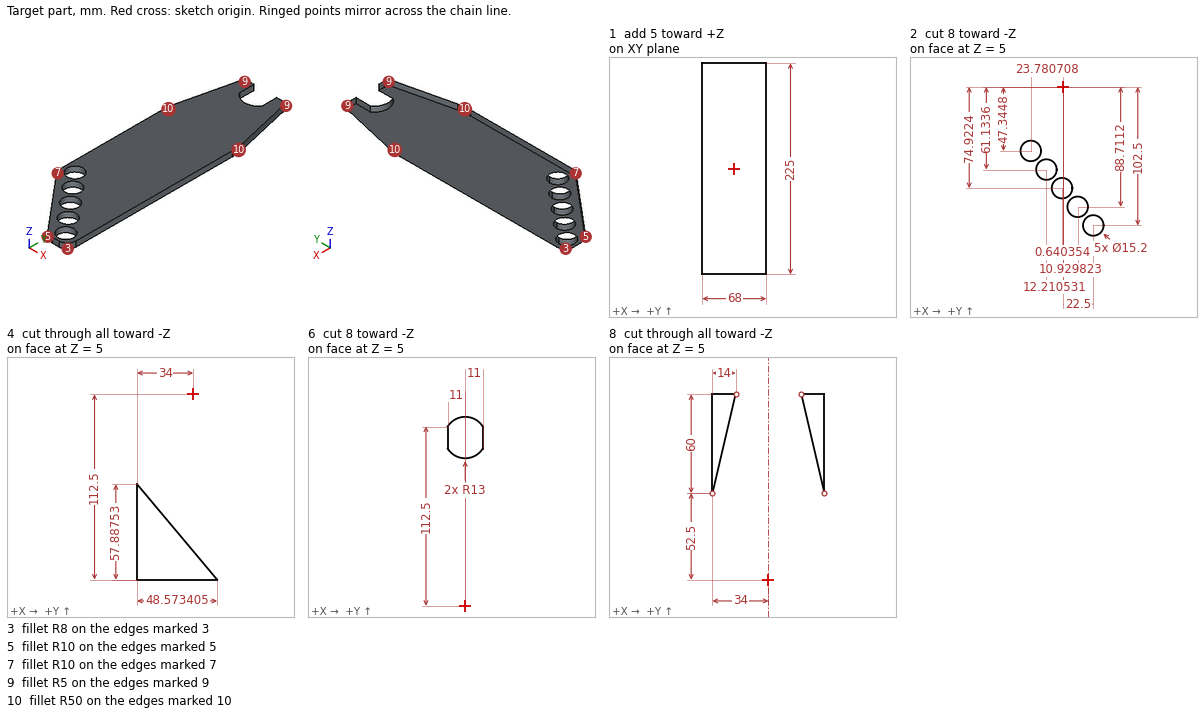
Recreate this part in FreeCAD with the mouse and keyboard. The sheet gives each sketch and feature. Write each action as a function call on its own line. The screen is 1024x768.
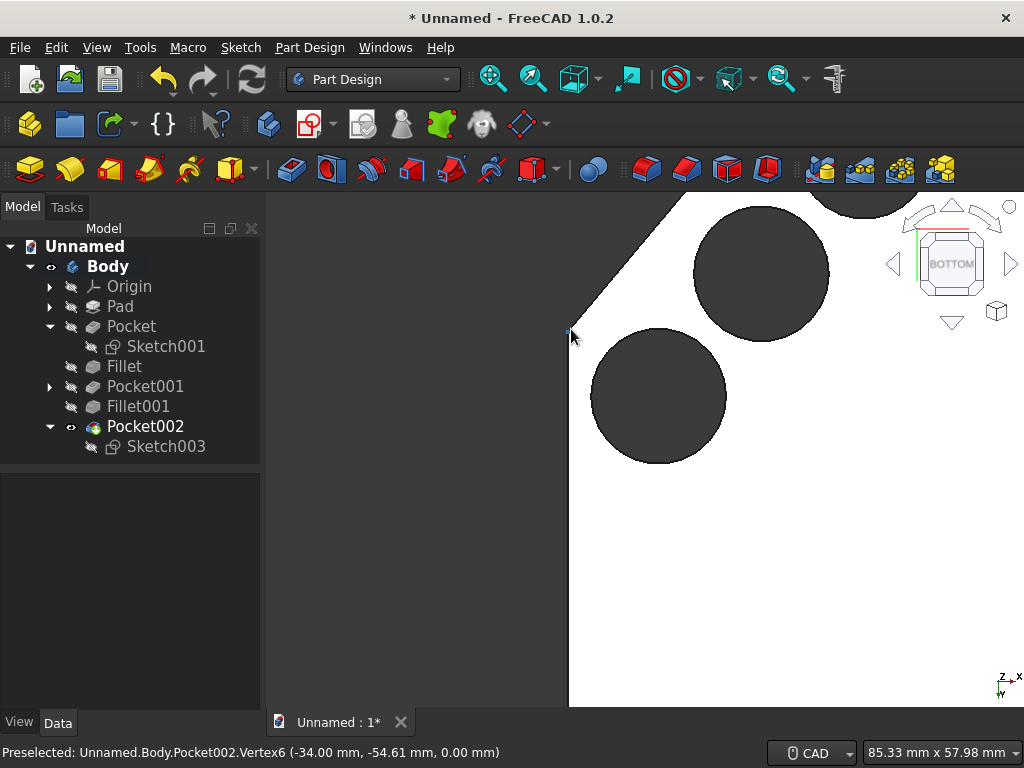
key(v)
key(f)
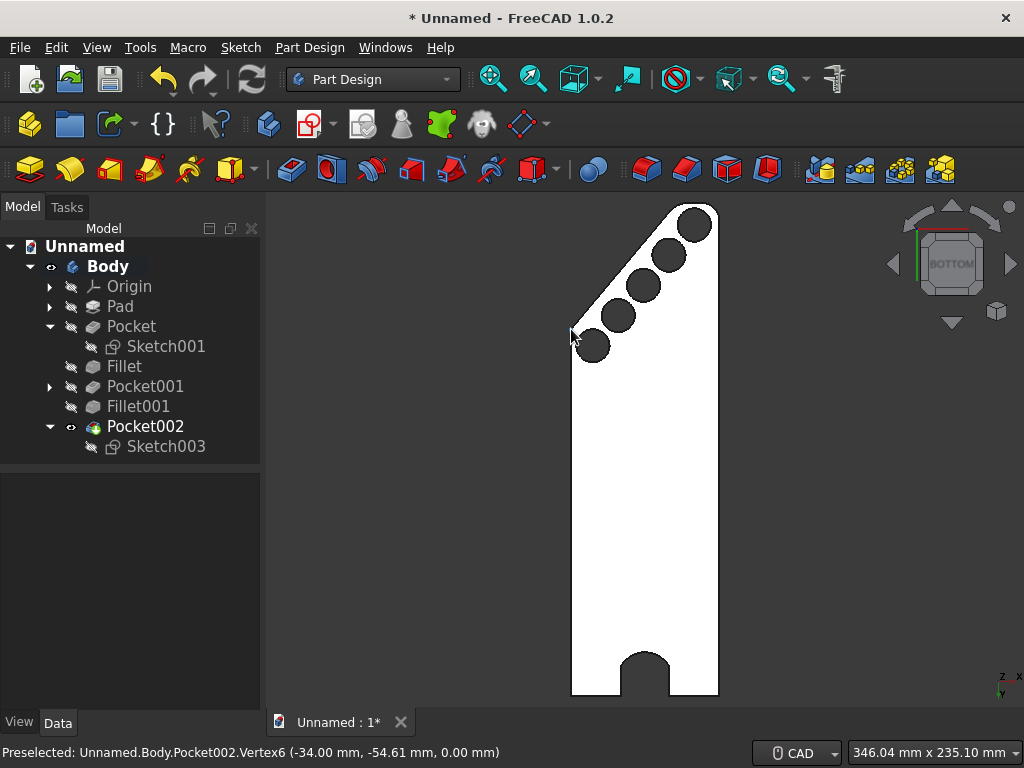
key(4)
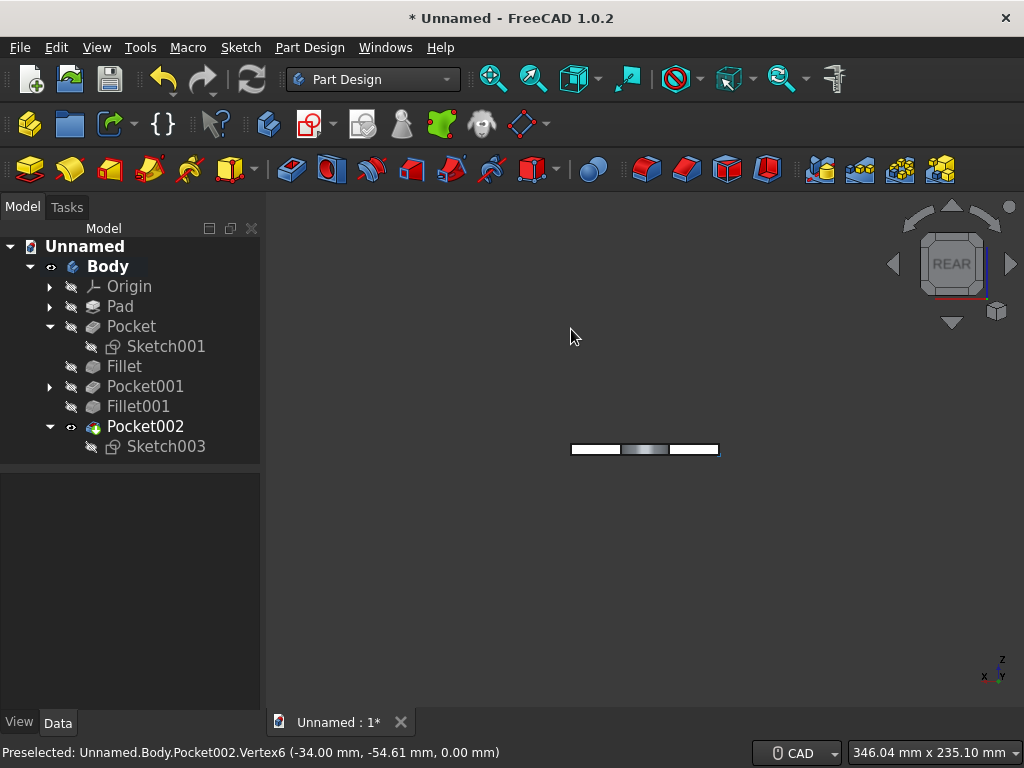
key(v)
key(f)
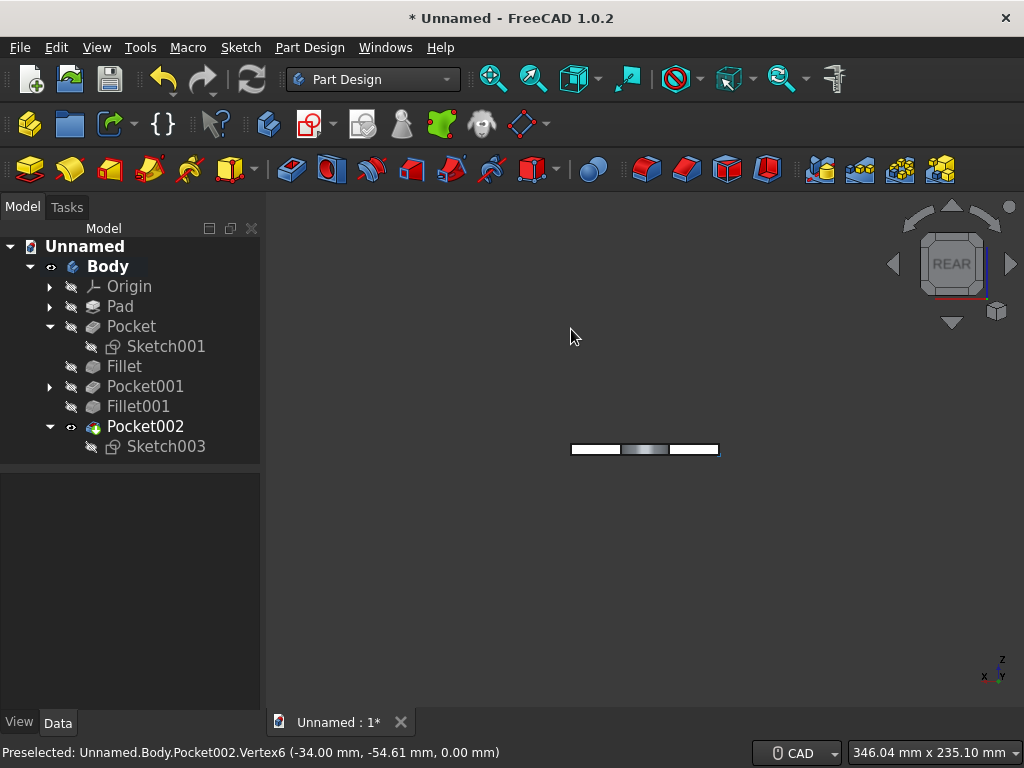
scroll(719, 449, up, 7)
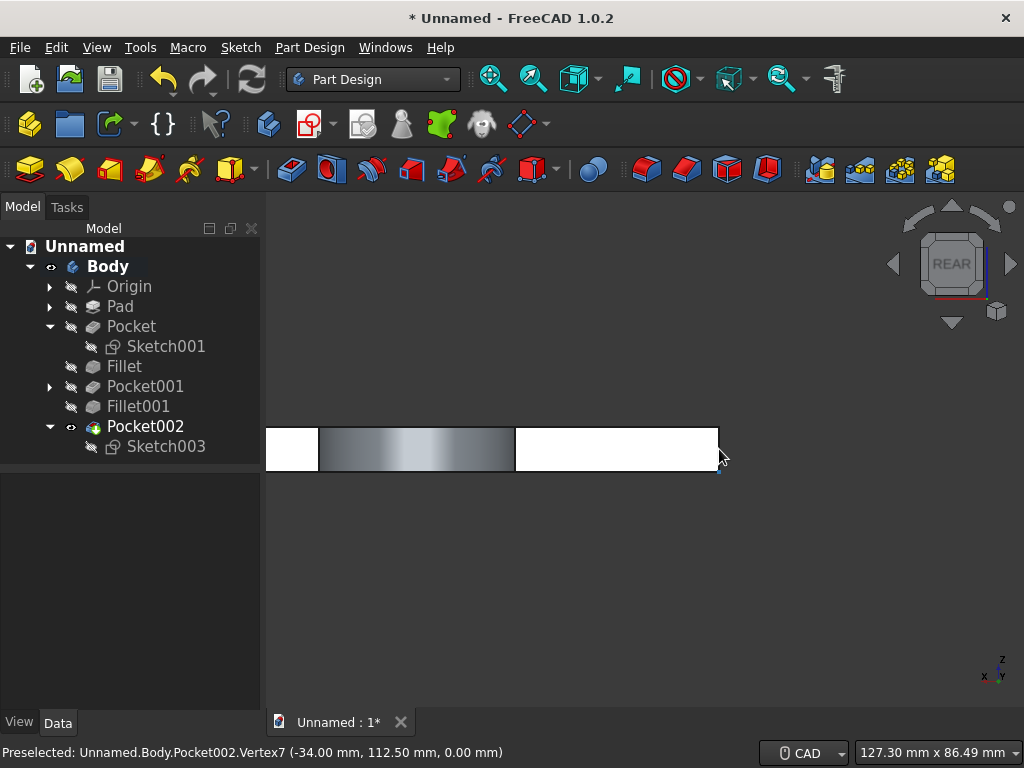
key(v)
key(f)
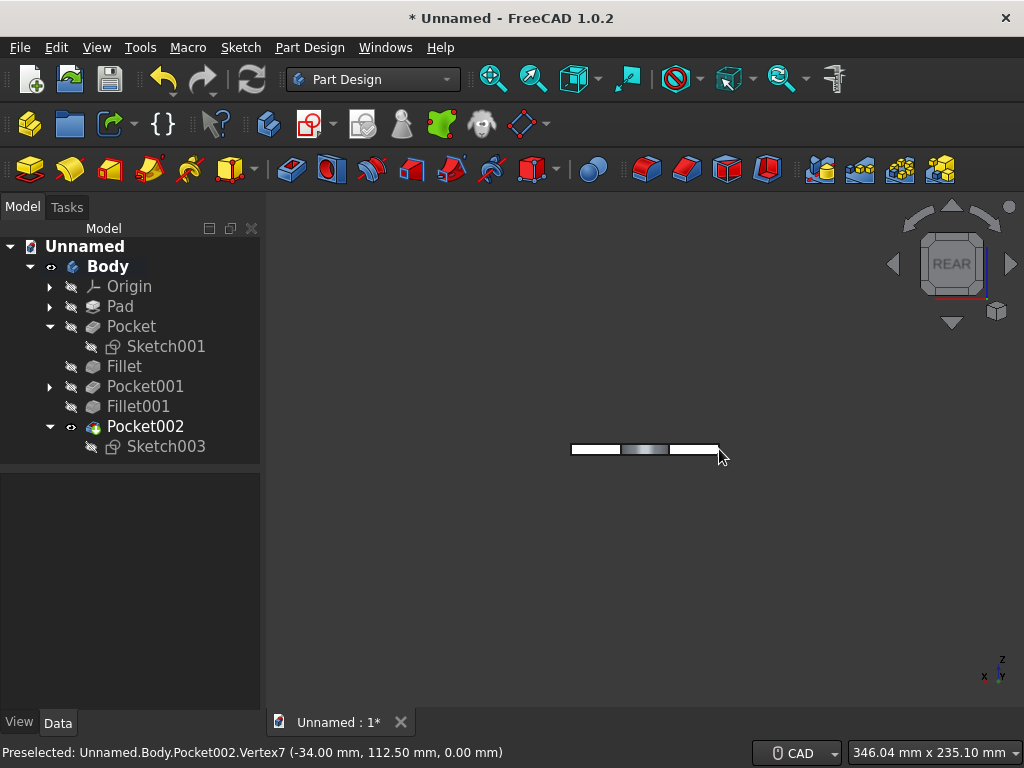
key(6)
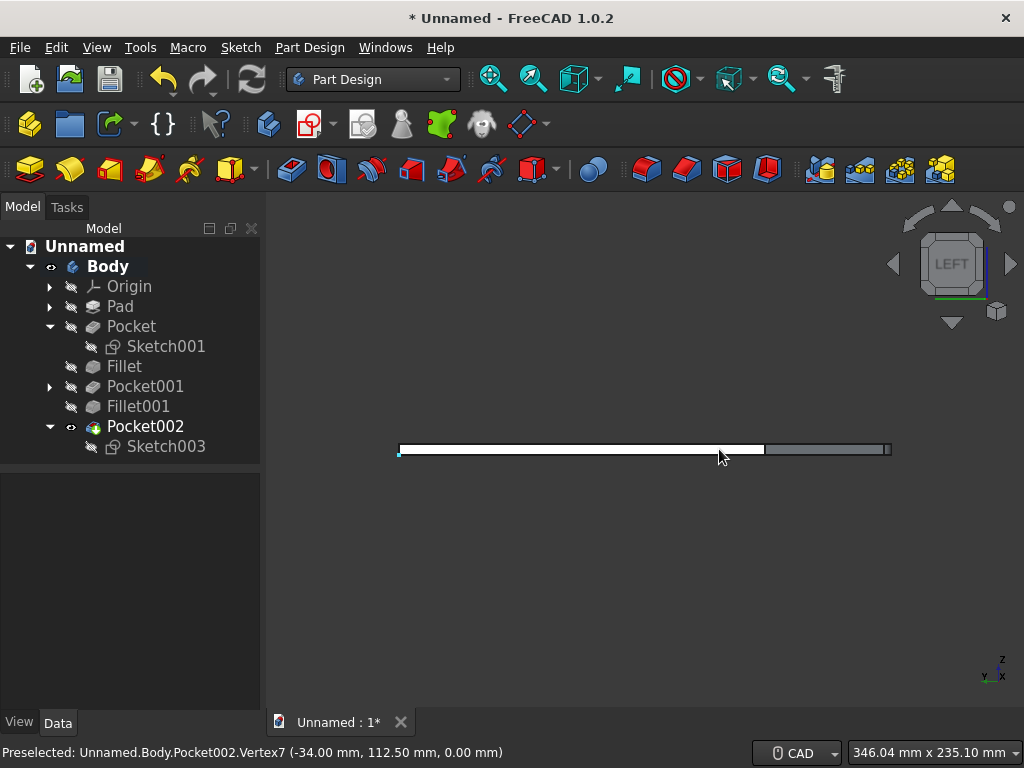
scroll(765, 448, up, 7)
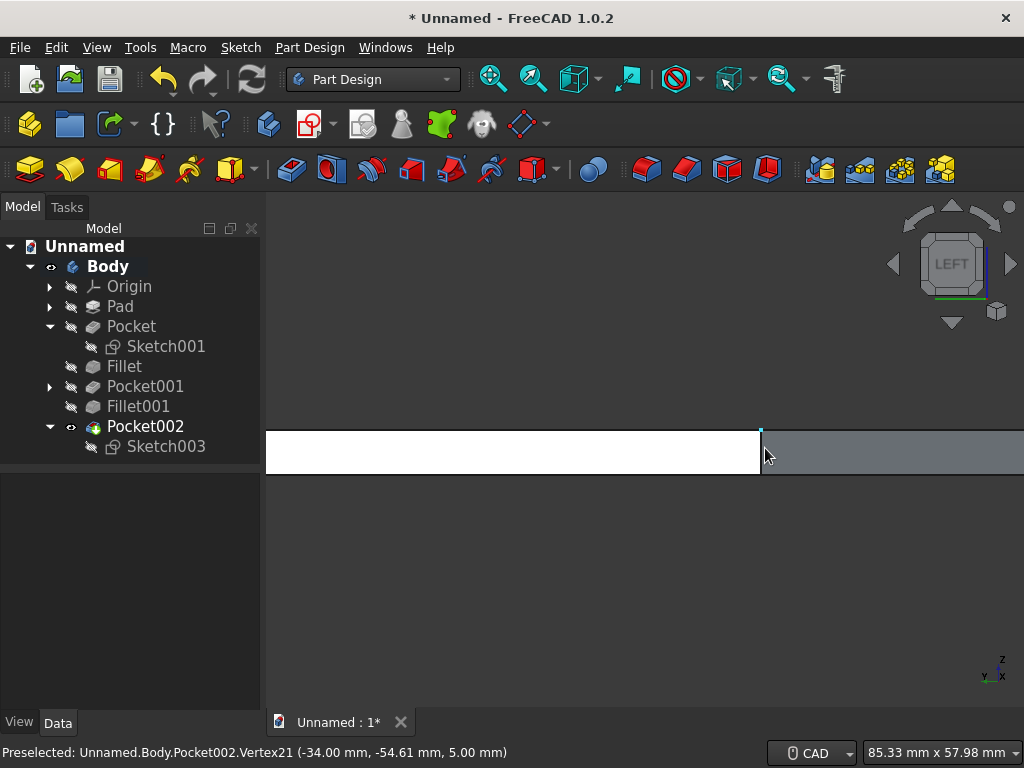
click(761, 452)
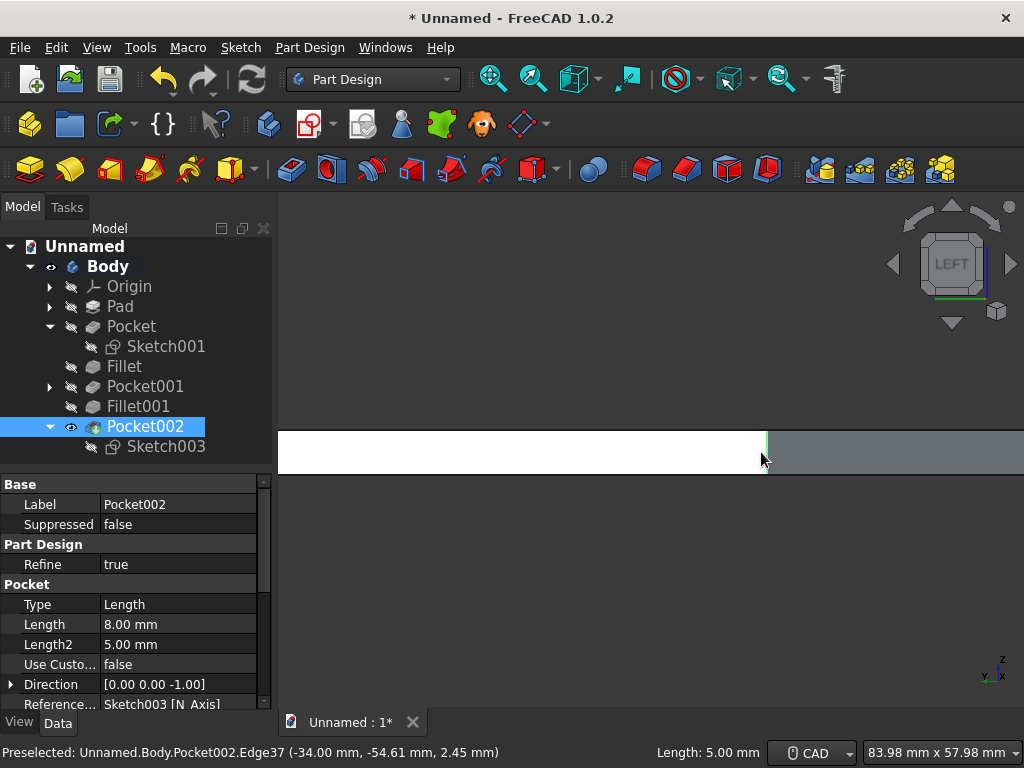
click(648, 170)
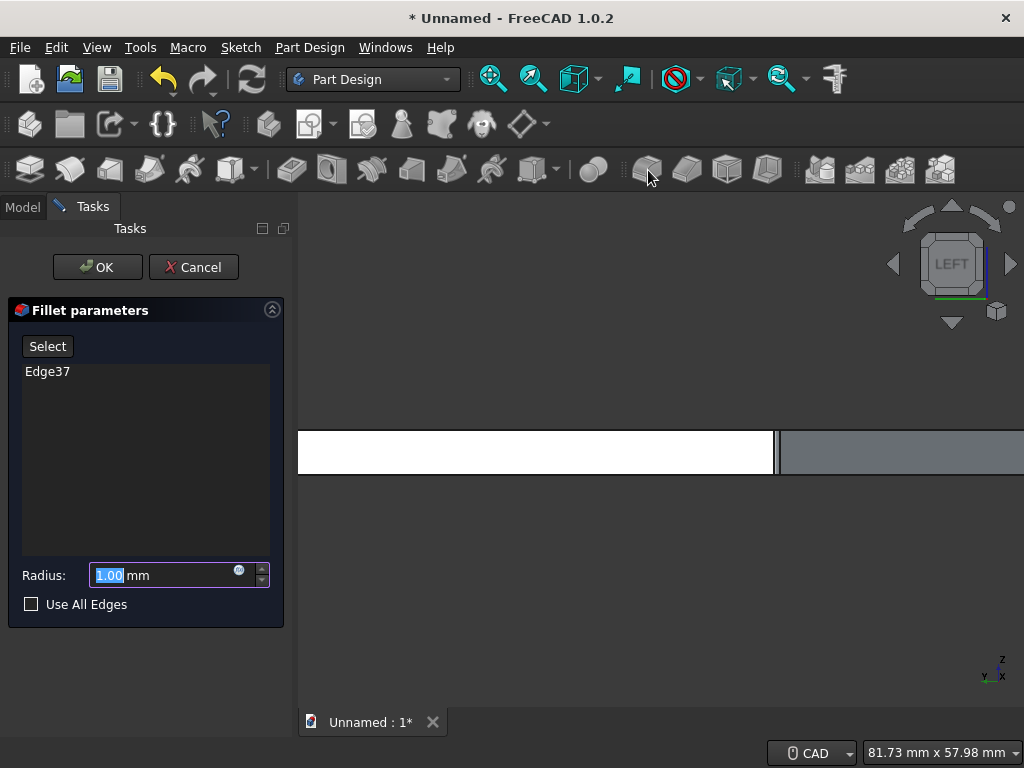
text(10)
key(Tab)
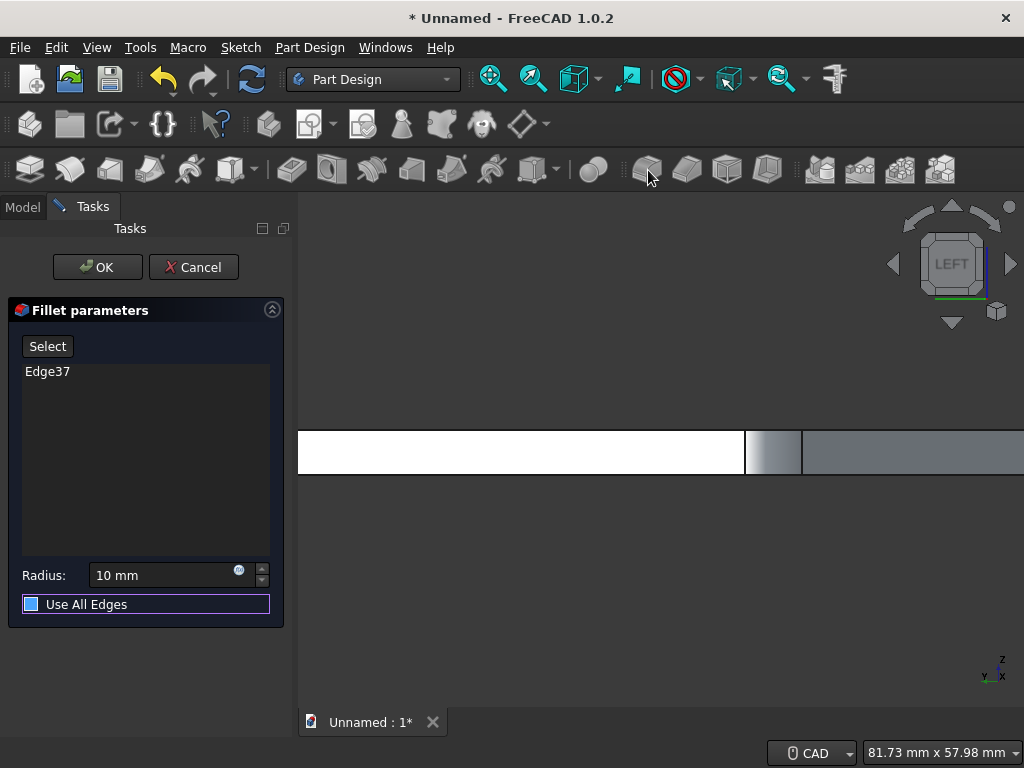
click(98, 267)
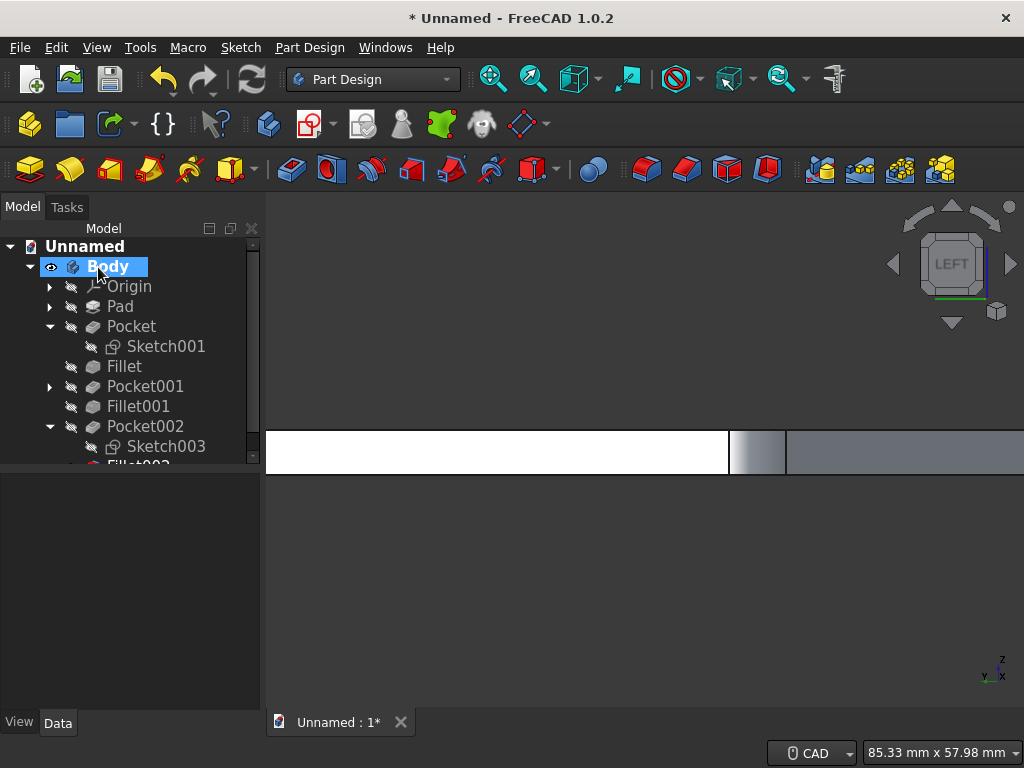
key(v)
key(f)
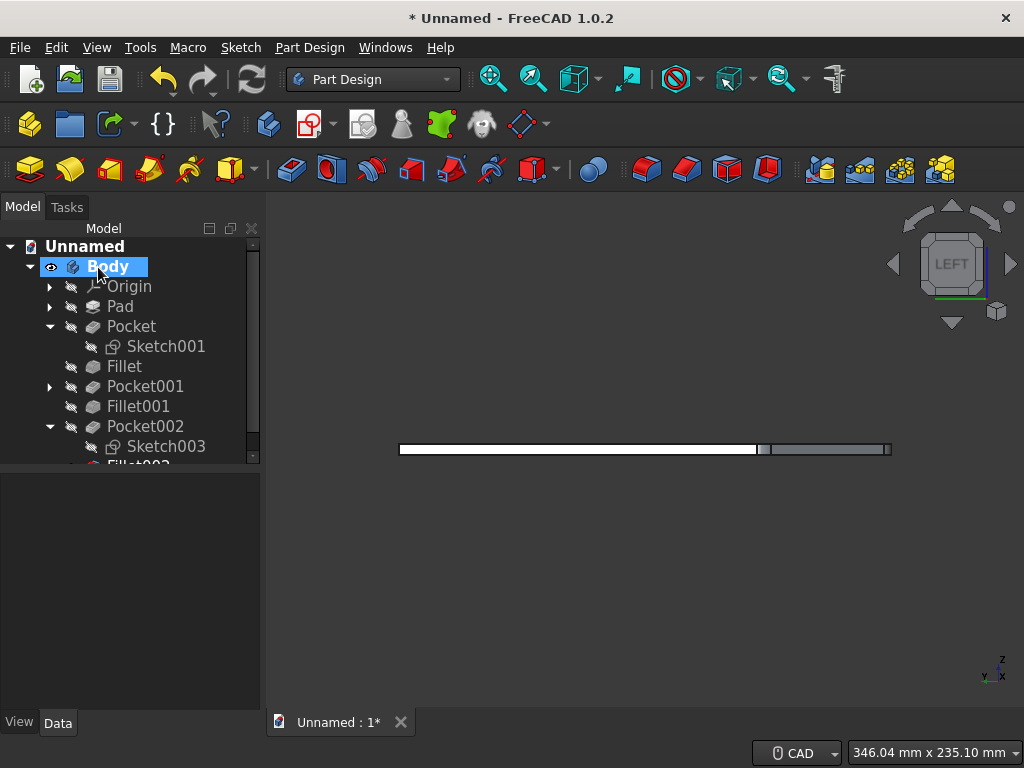
key(0)